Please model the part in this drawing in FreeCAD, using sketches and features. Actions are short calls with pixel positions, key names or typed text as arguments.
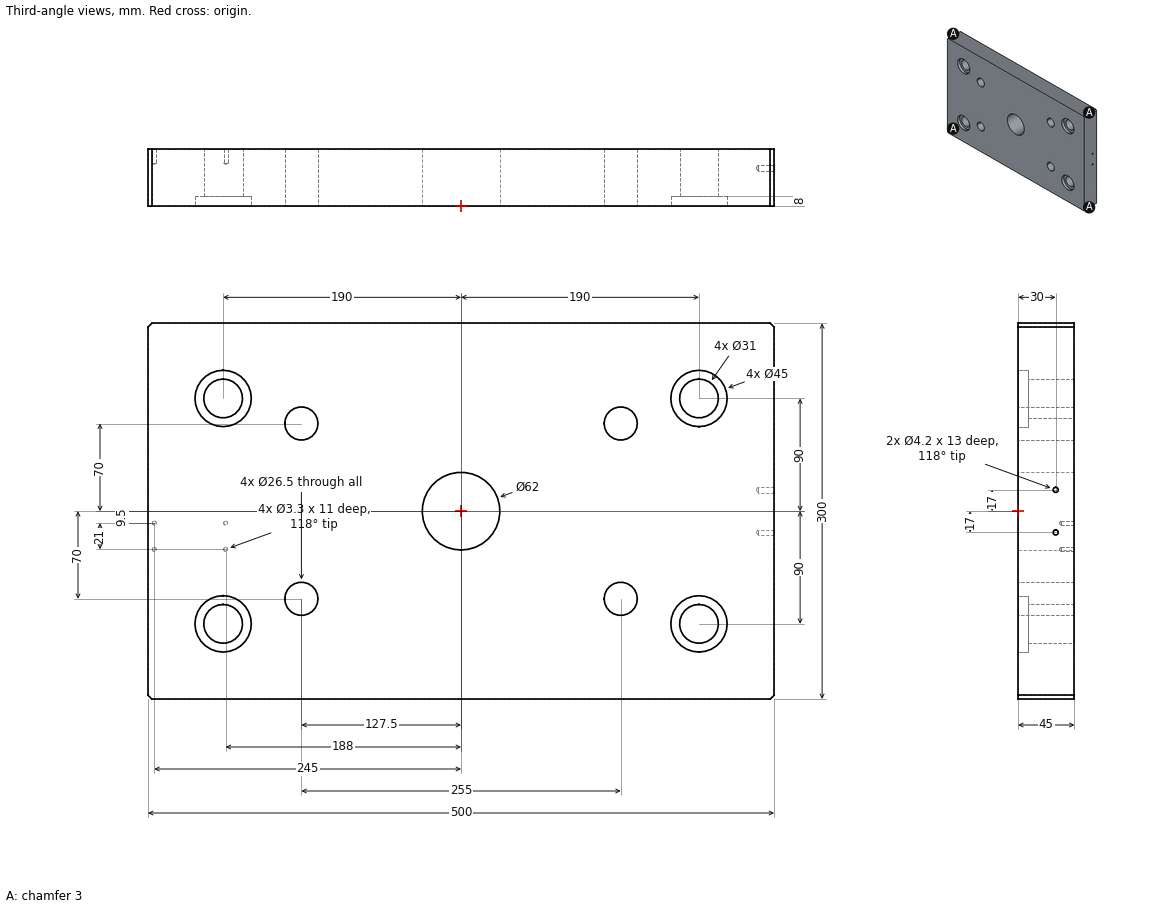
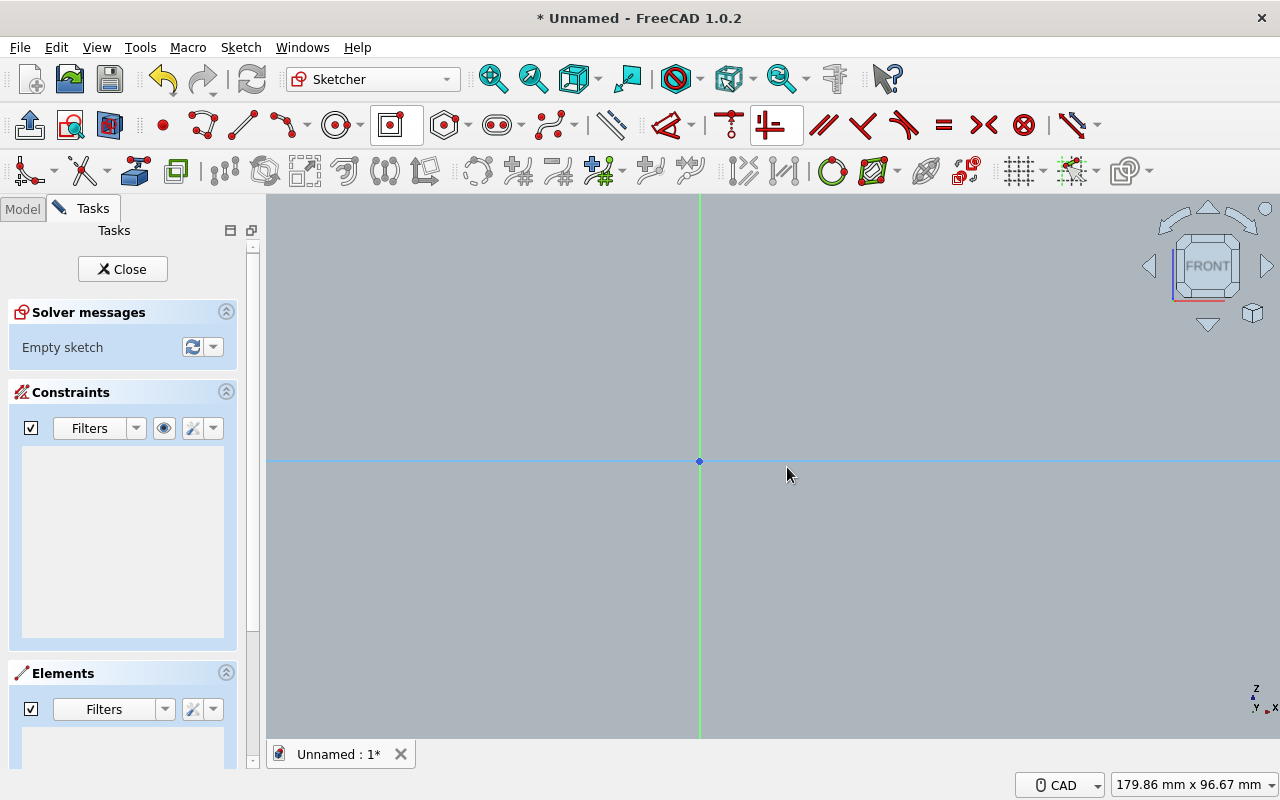
click(336, 126)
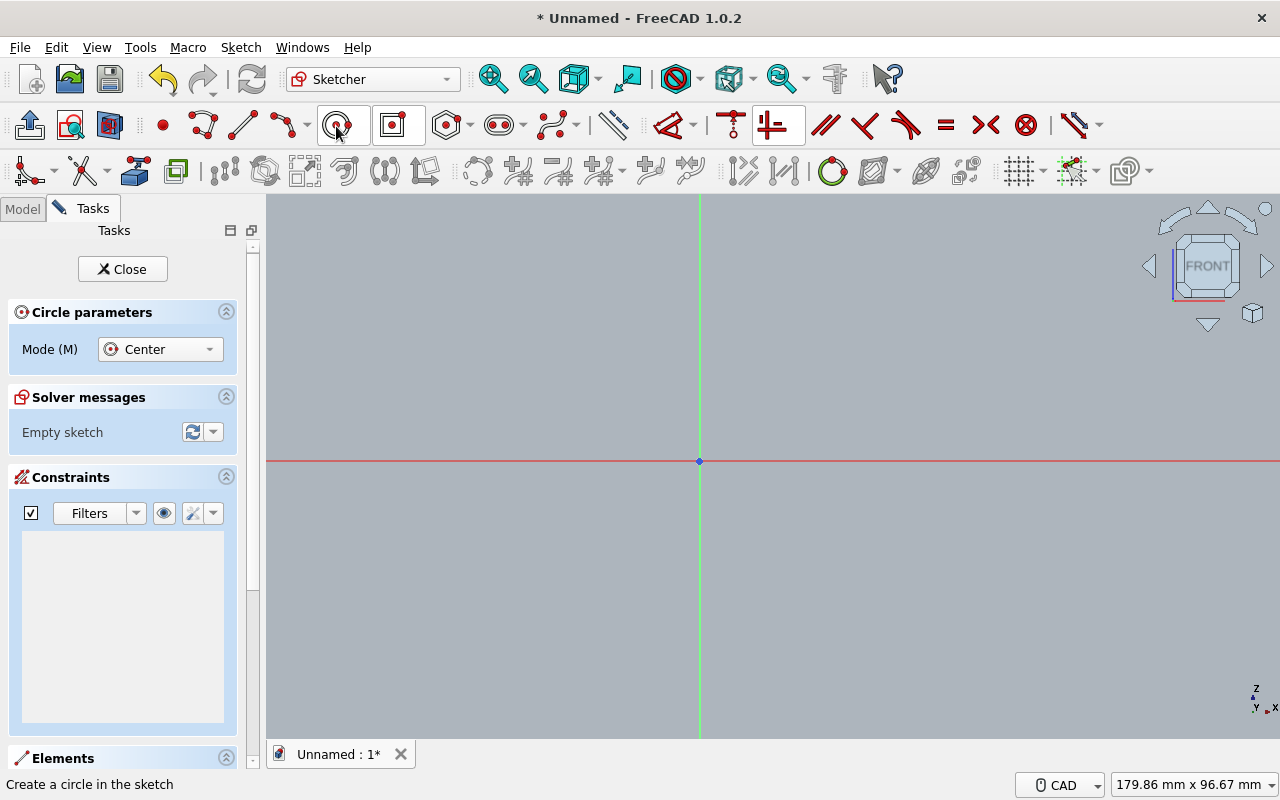
click(700, 461)
click(823, 338)
key(Escape)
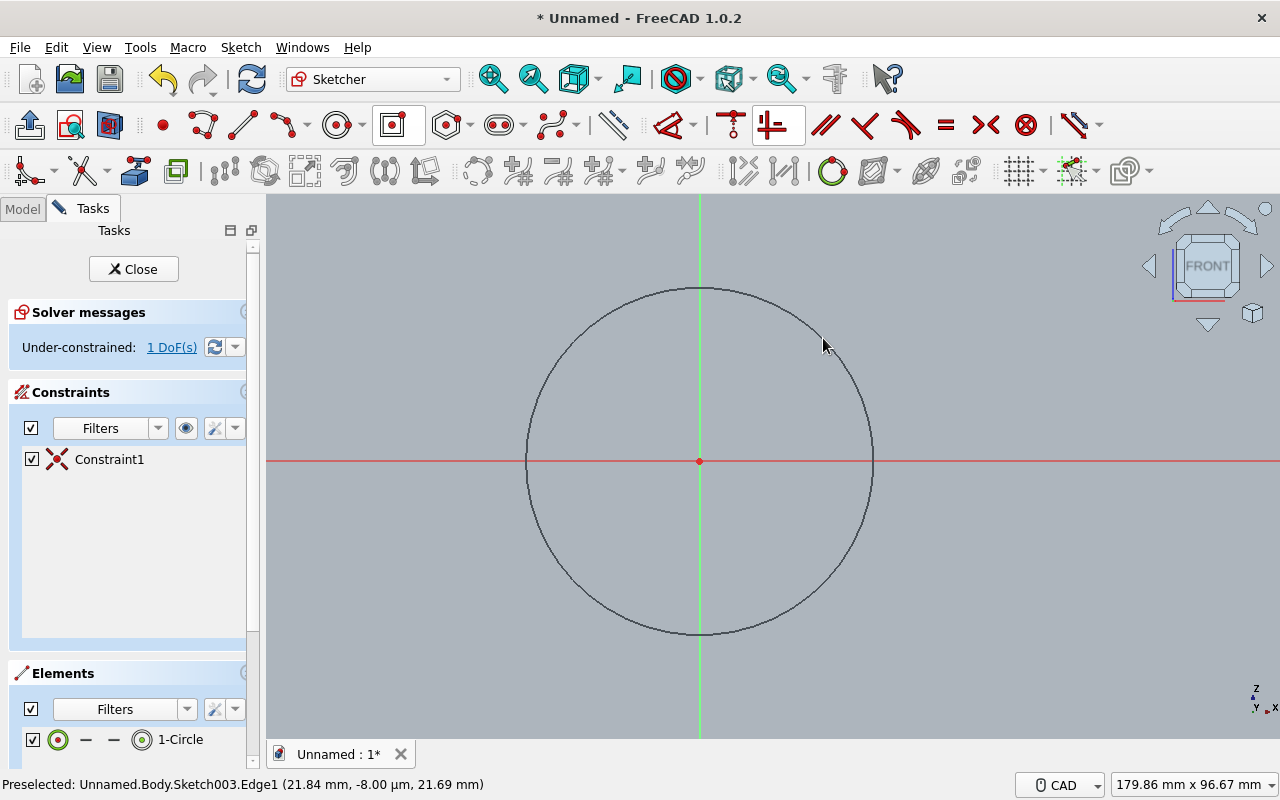
click(668, 126)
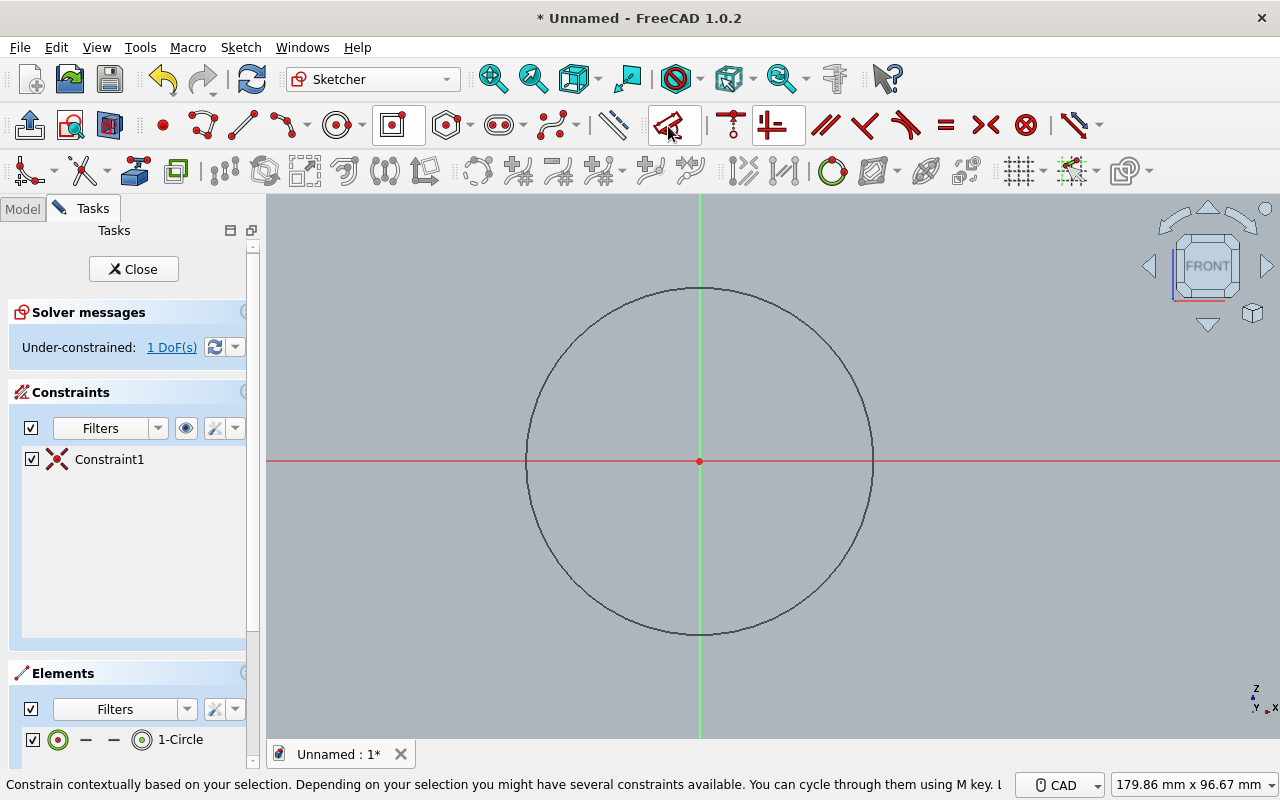
click(822, 338)
click(845, 315)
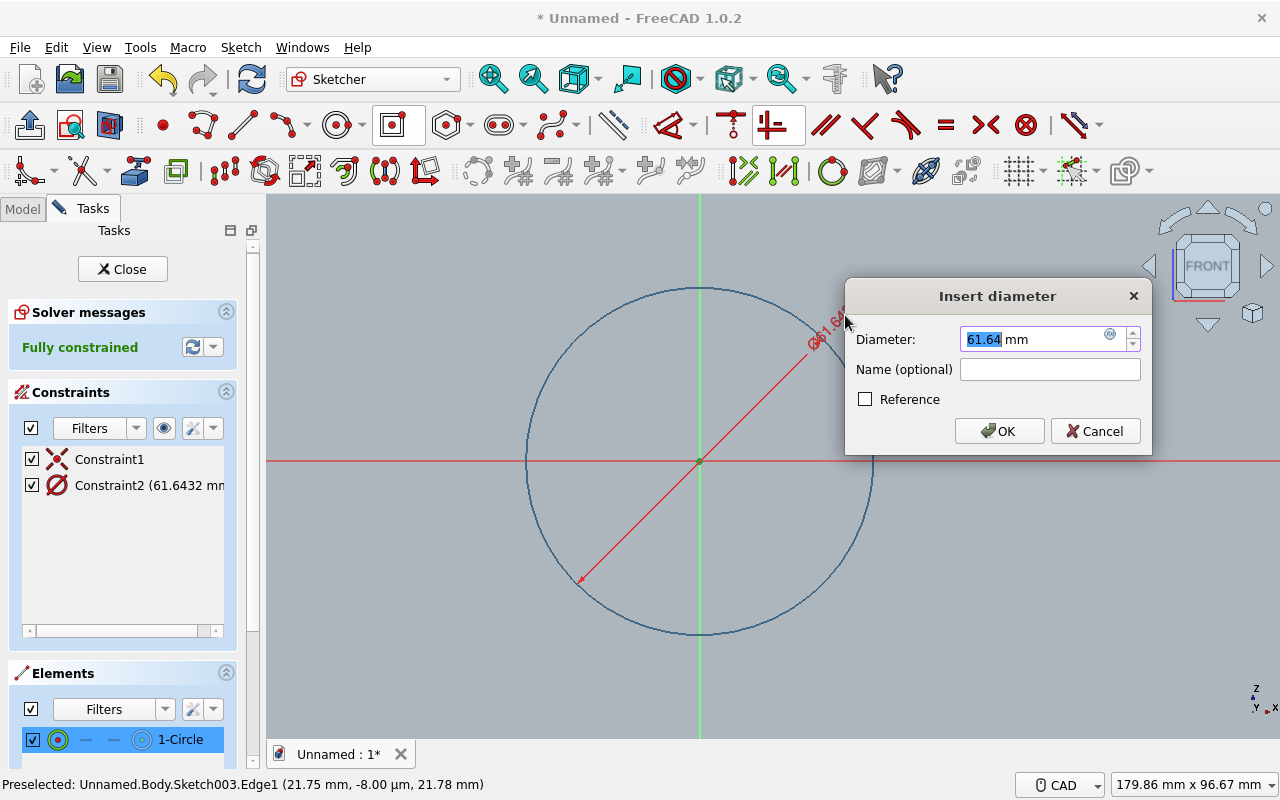
text(62)
key(Return)
key(Escape)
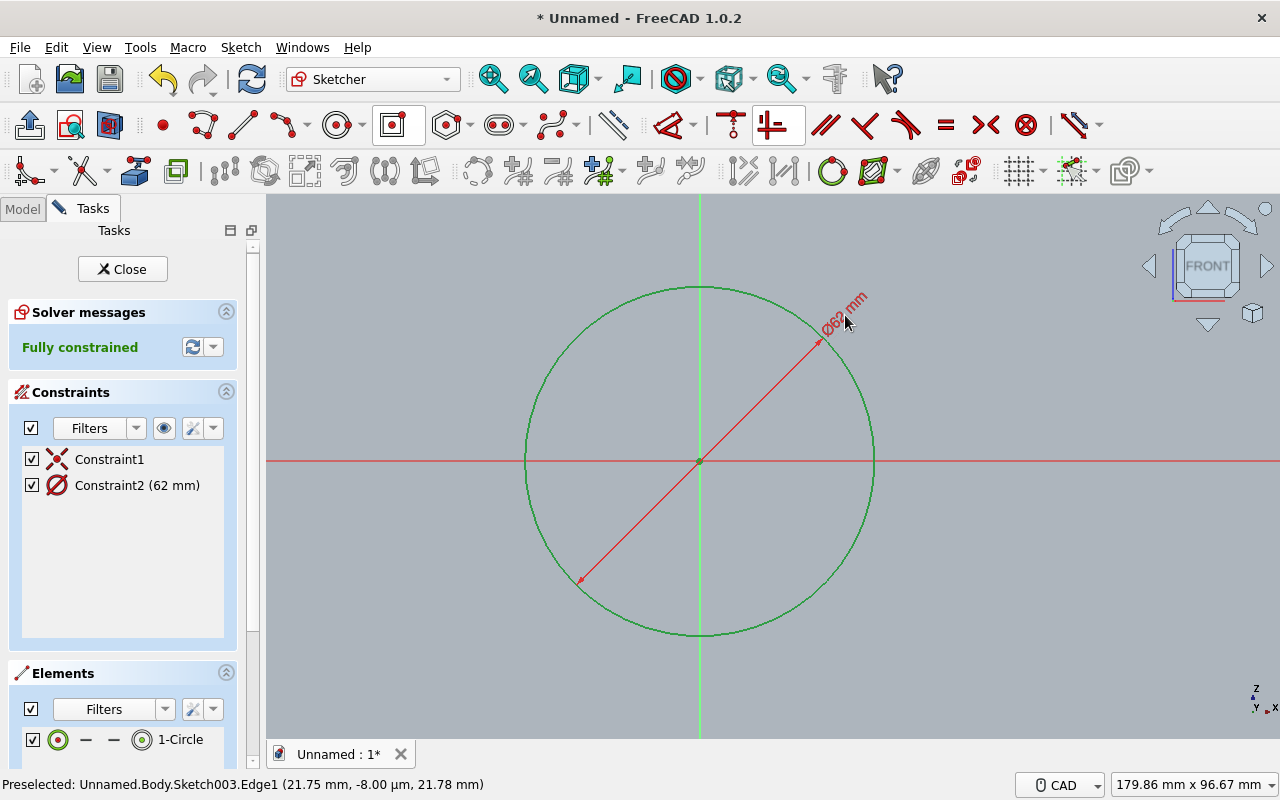
click(123, 269)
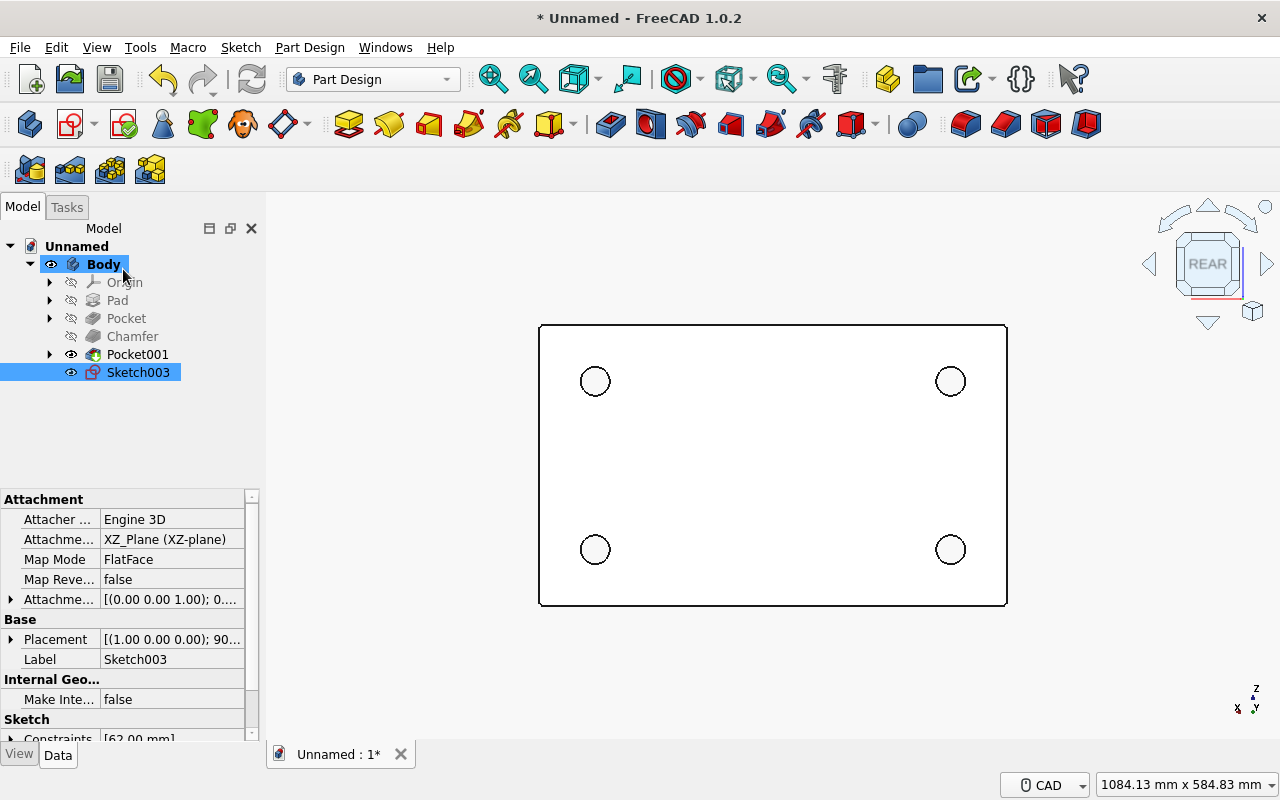
click(612, 124)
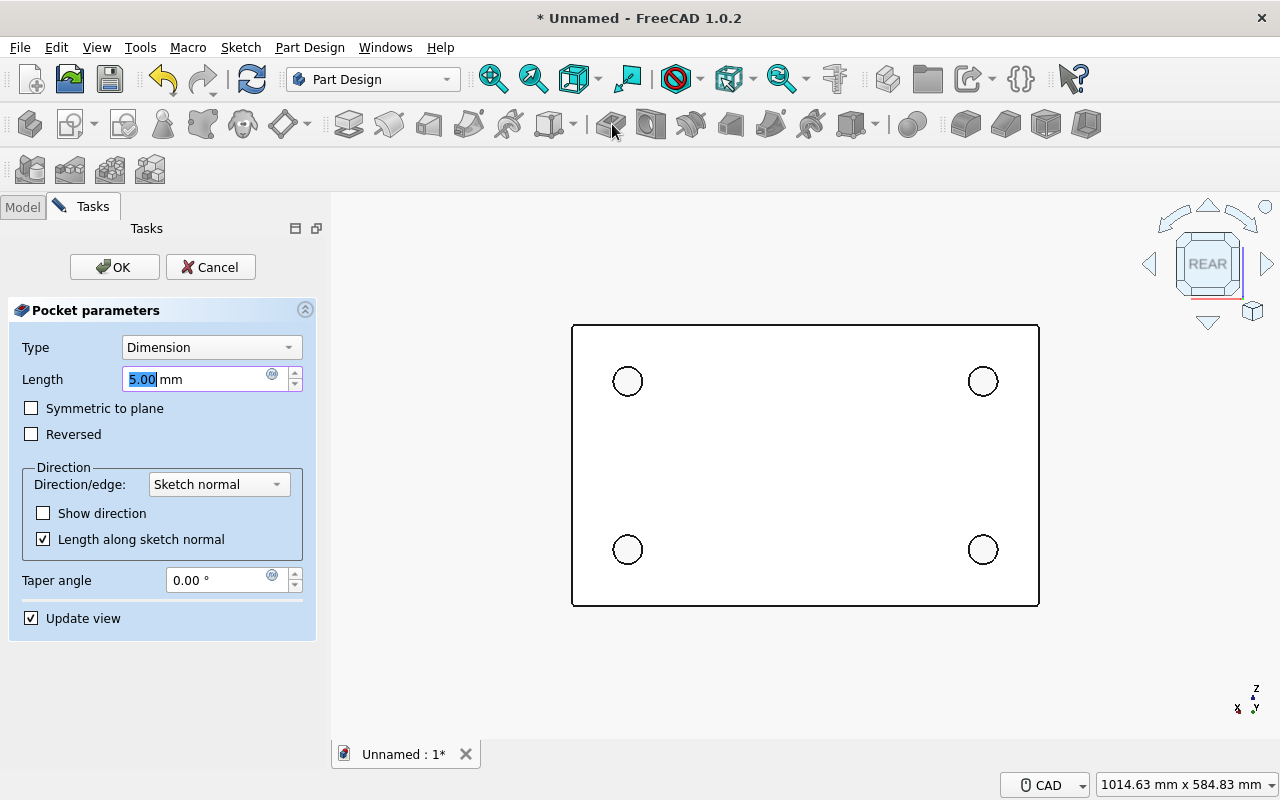
click(212, 348)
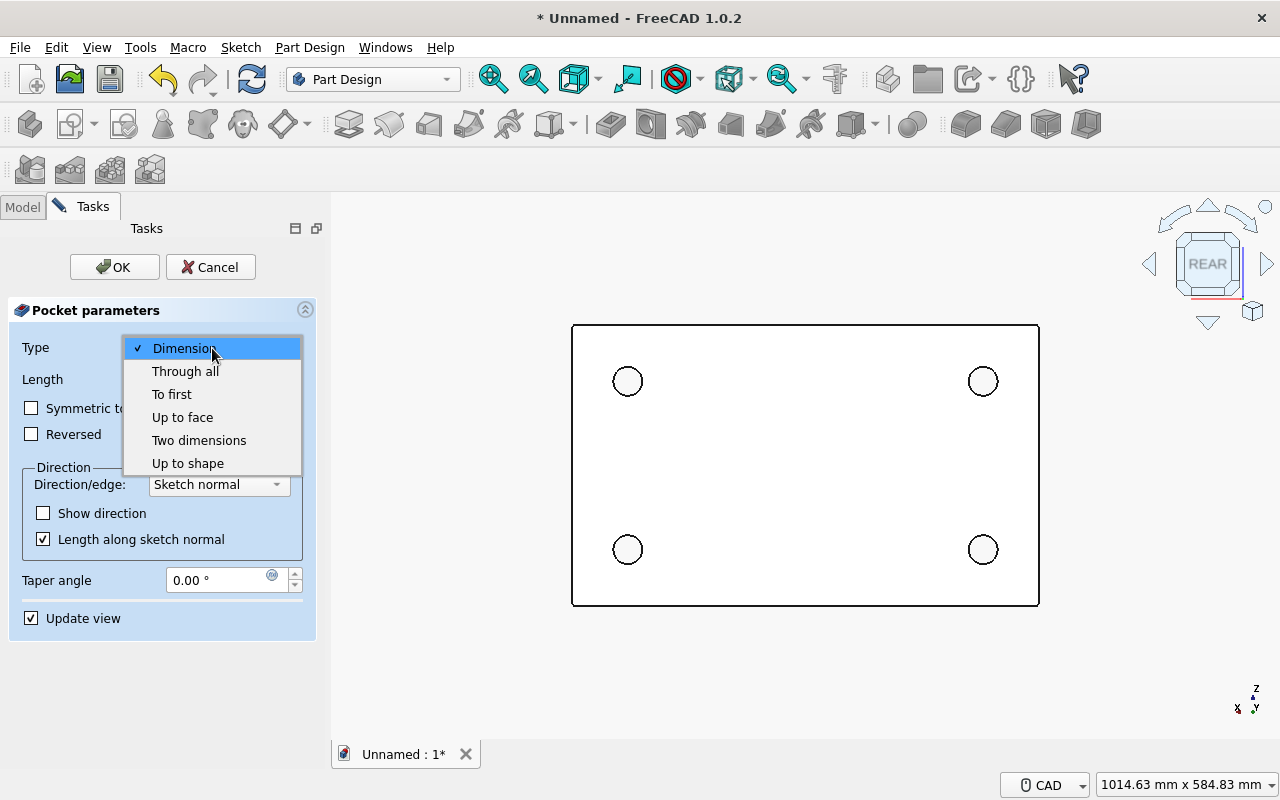
click(212, 372)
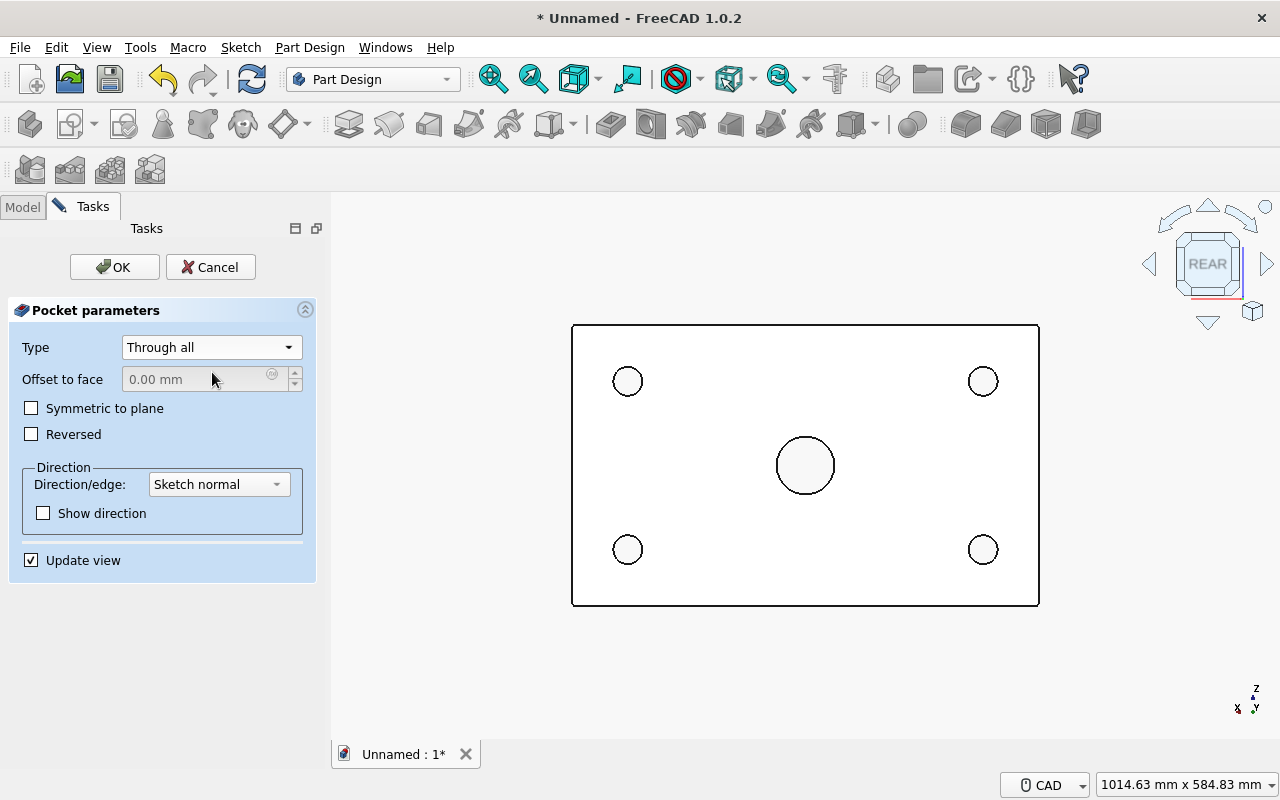
click(115, 267)